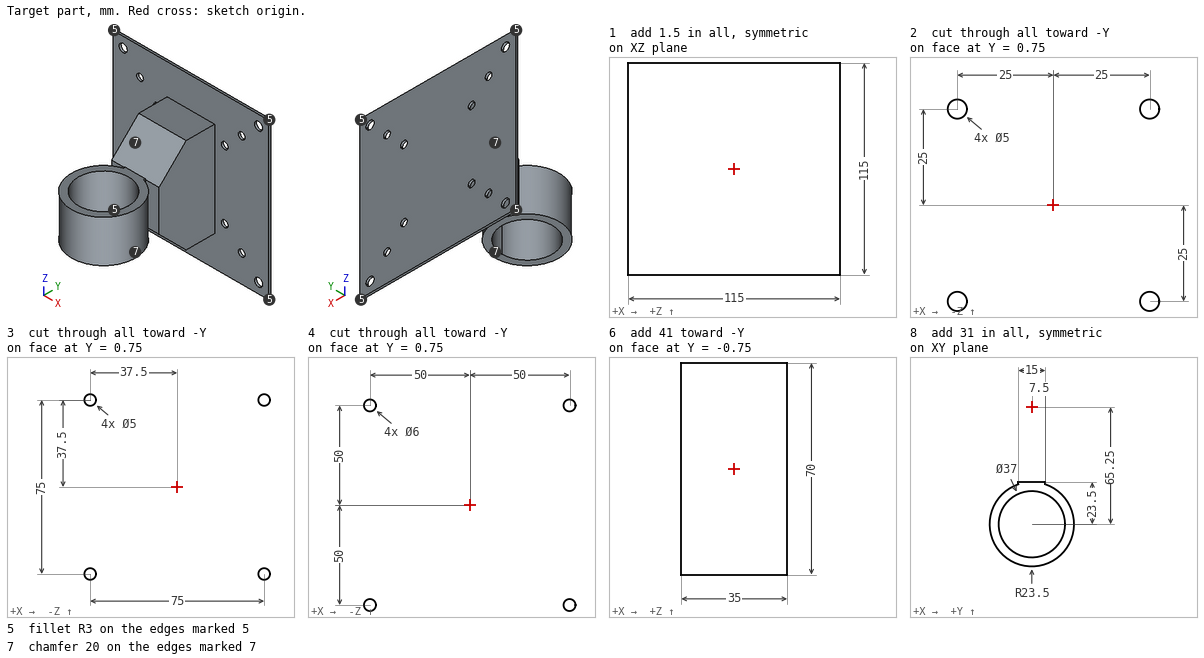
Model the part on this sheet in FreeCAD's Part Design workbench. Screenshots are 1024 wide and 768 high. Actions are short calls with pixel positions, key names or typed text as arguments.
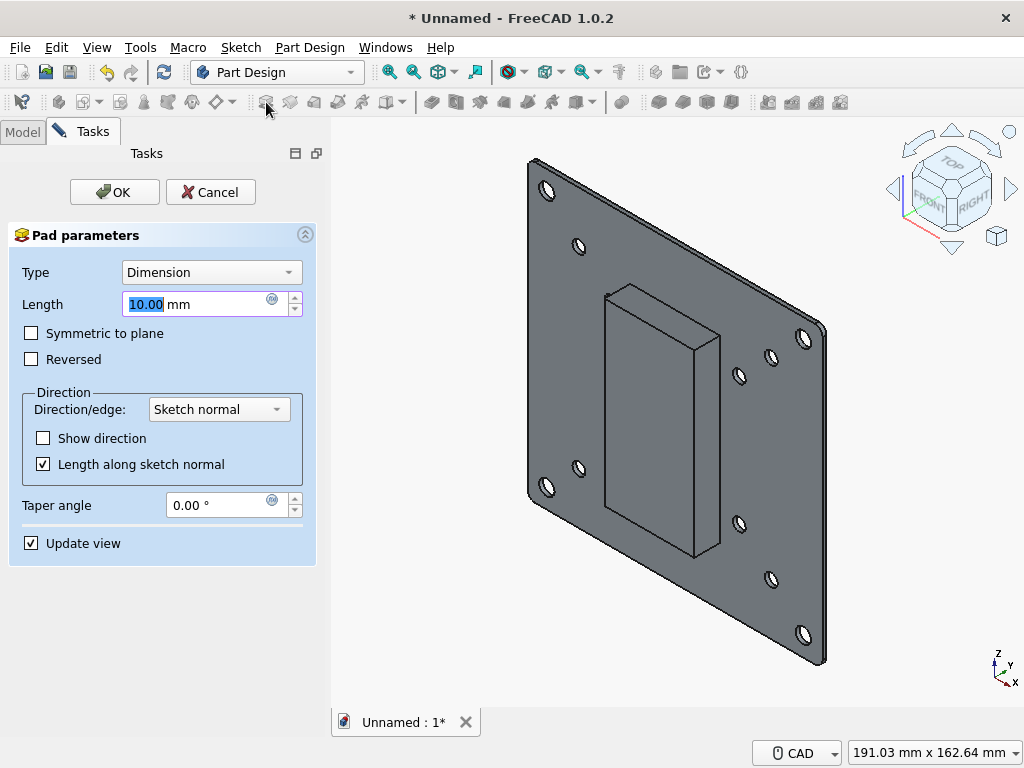
text(41)
key(Tab)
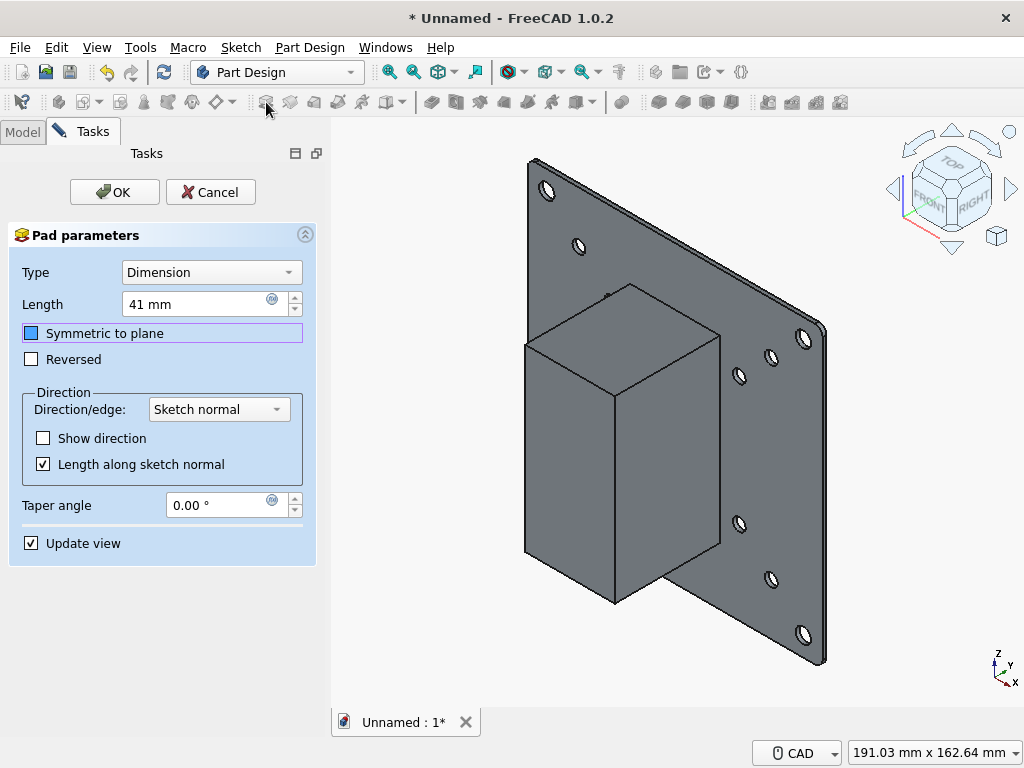
click(115, 192)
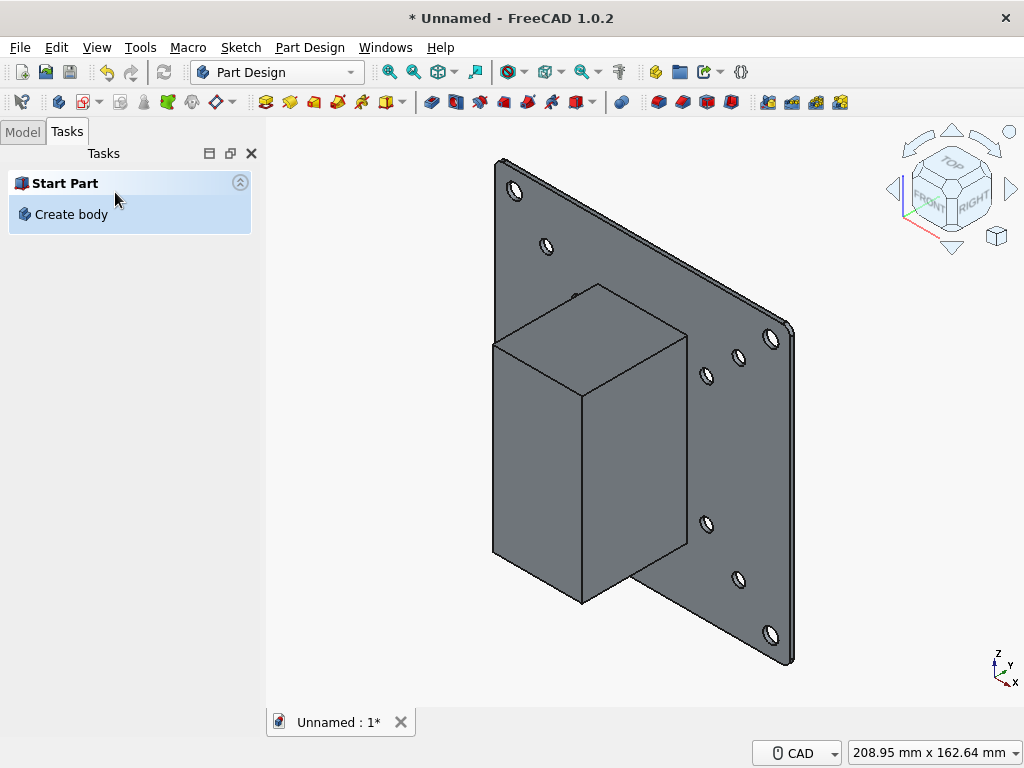
key(v)
key(f)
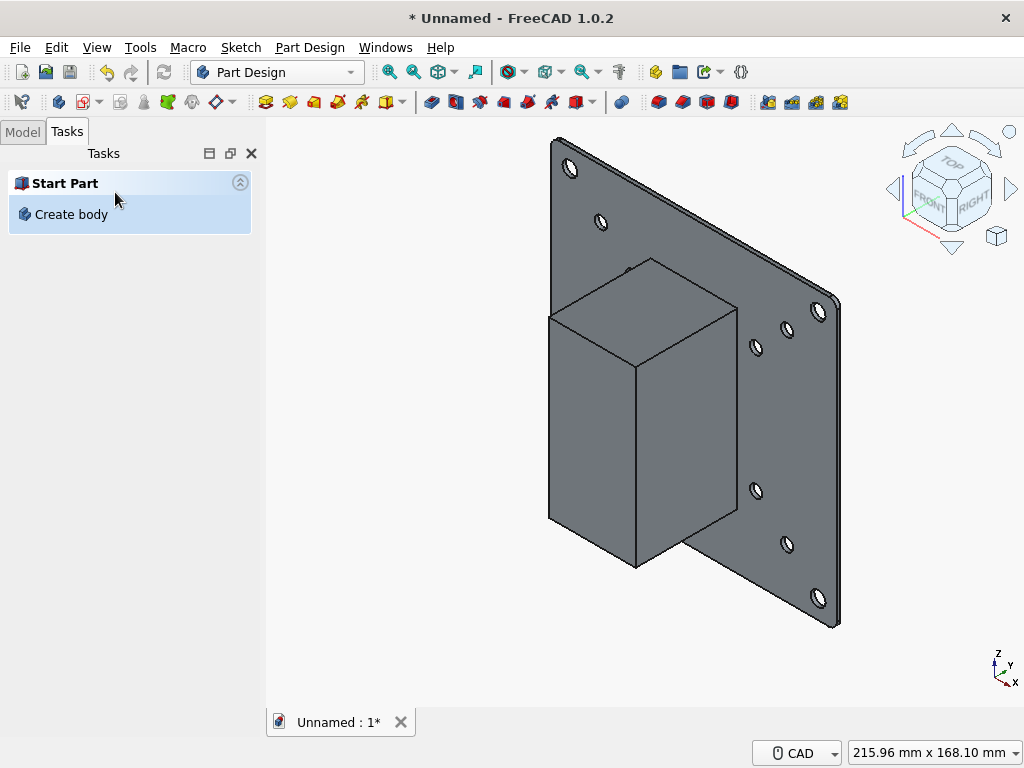
click(592, 341)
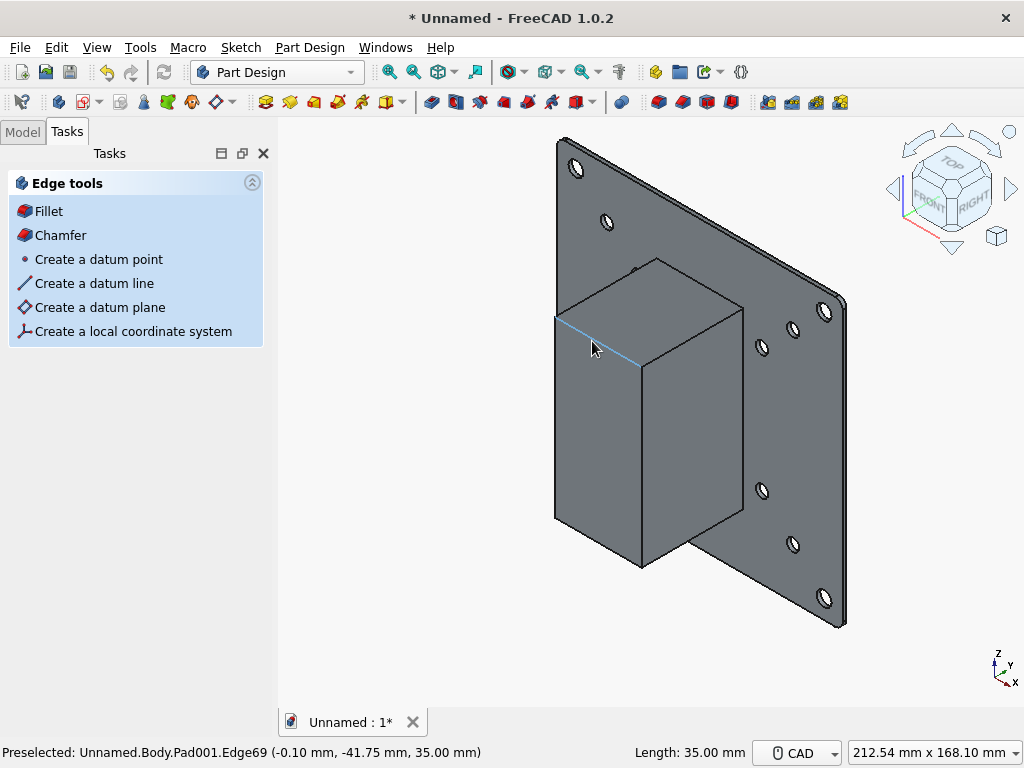
key(2)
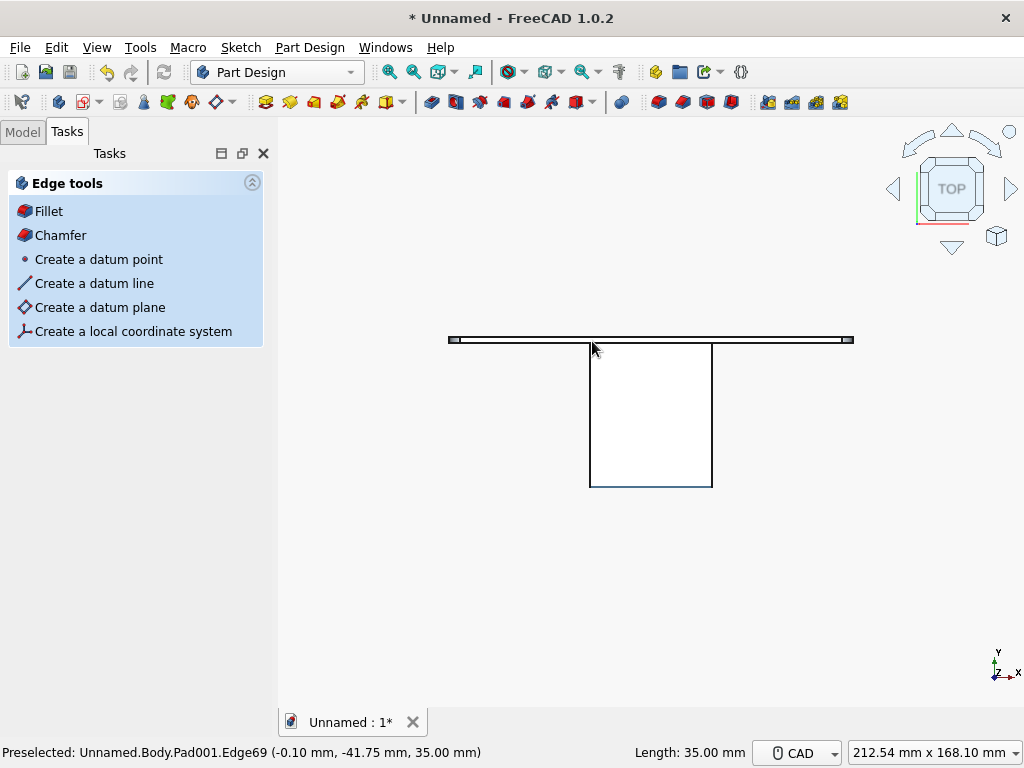
key(0)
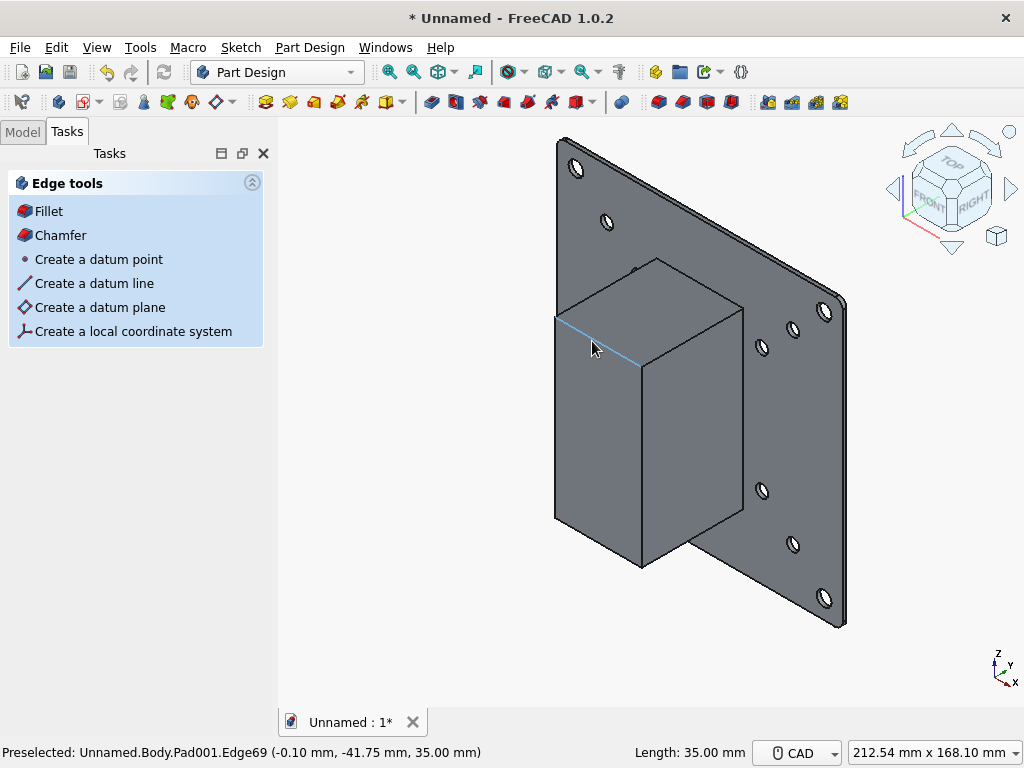
key(1)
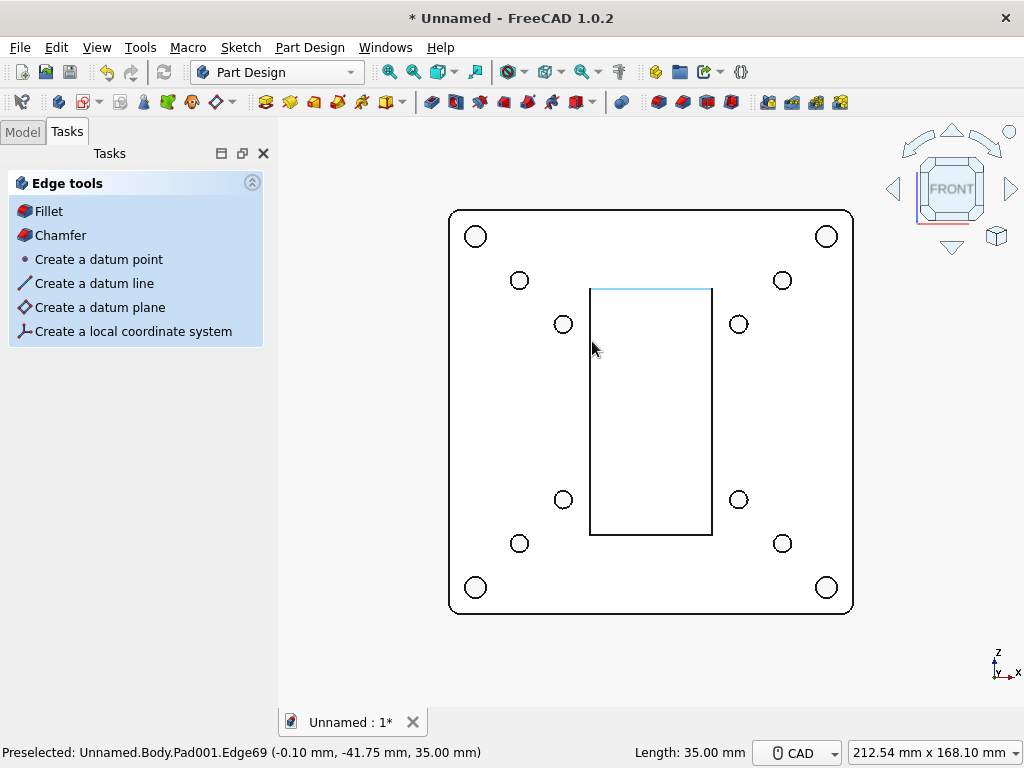
key(3)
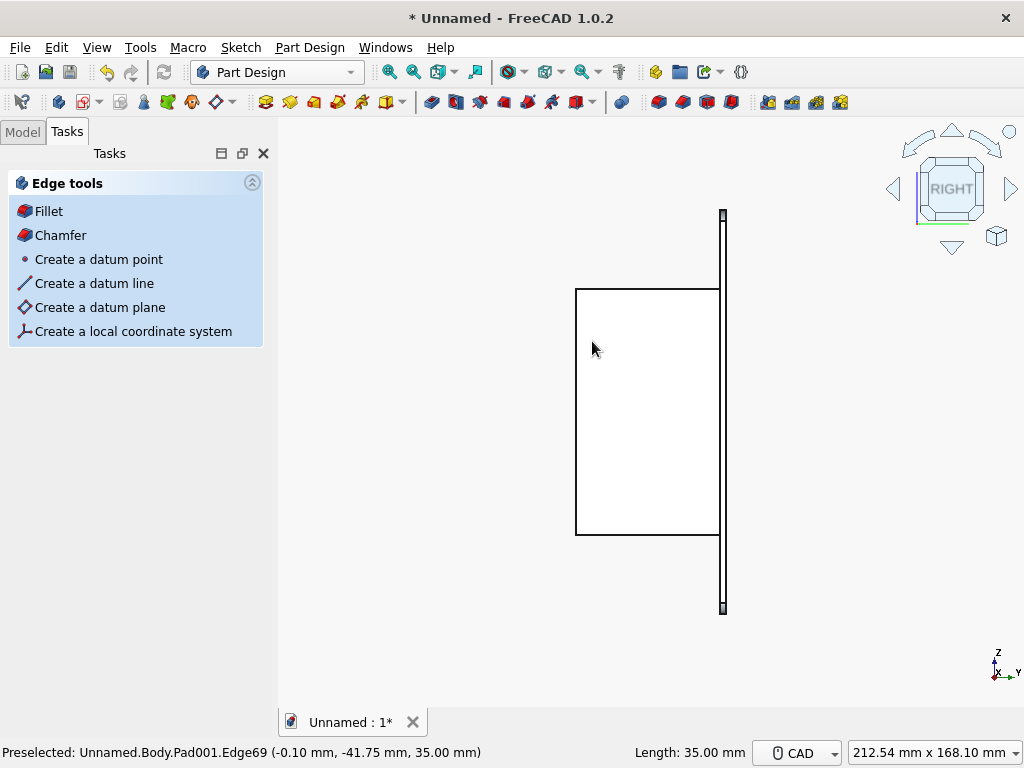
key(5)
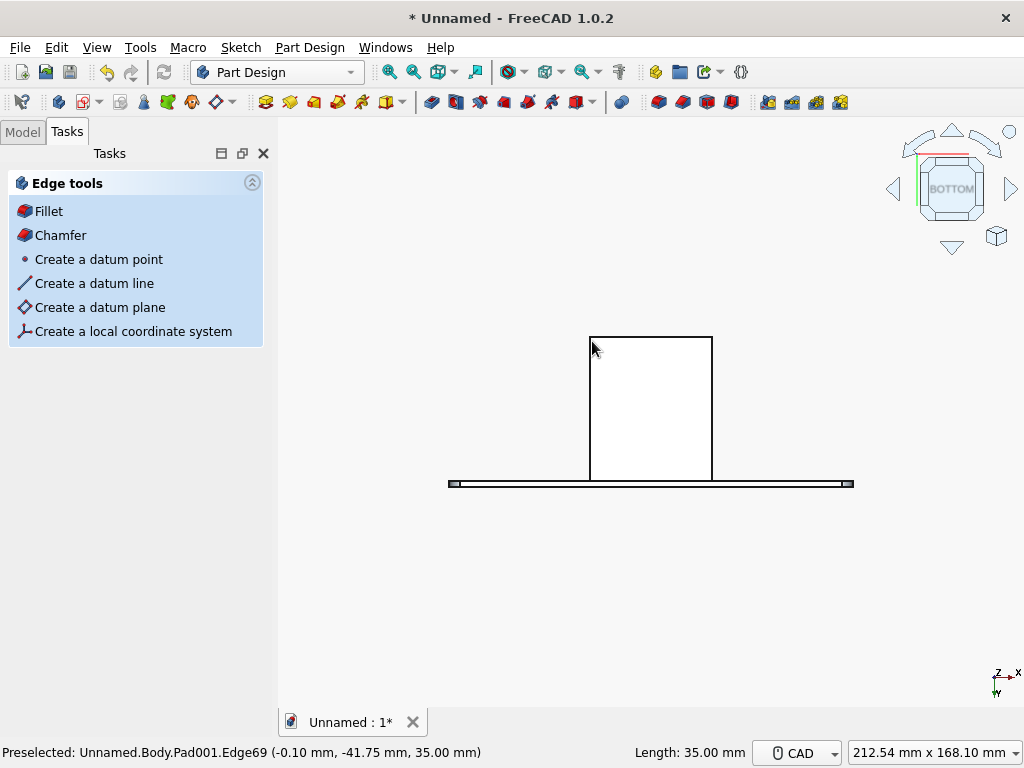
click(651, 336, ctrl)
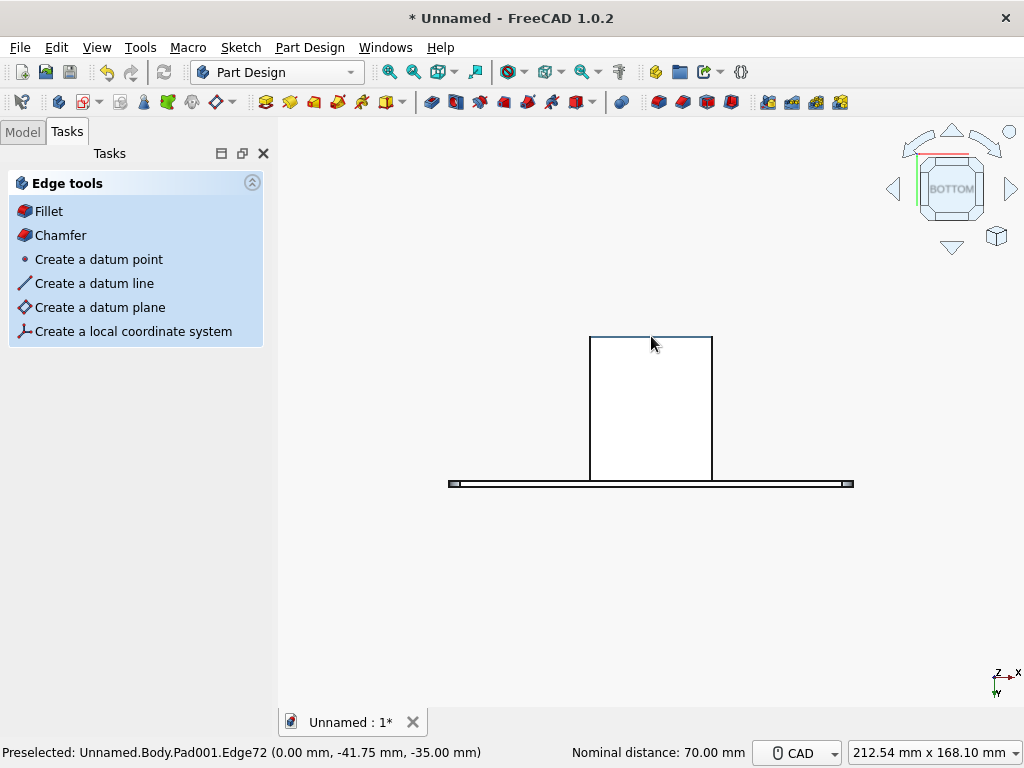
click(684, 102)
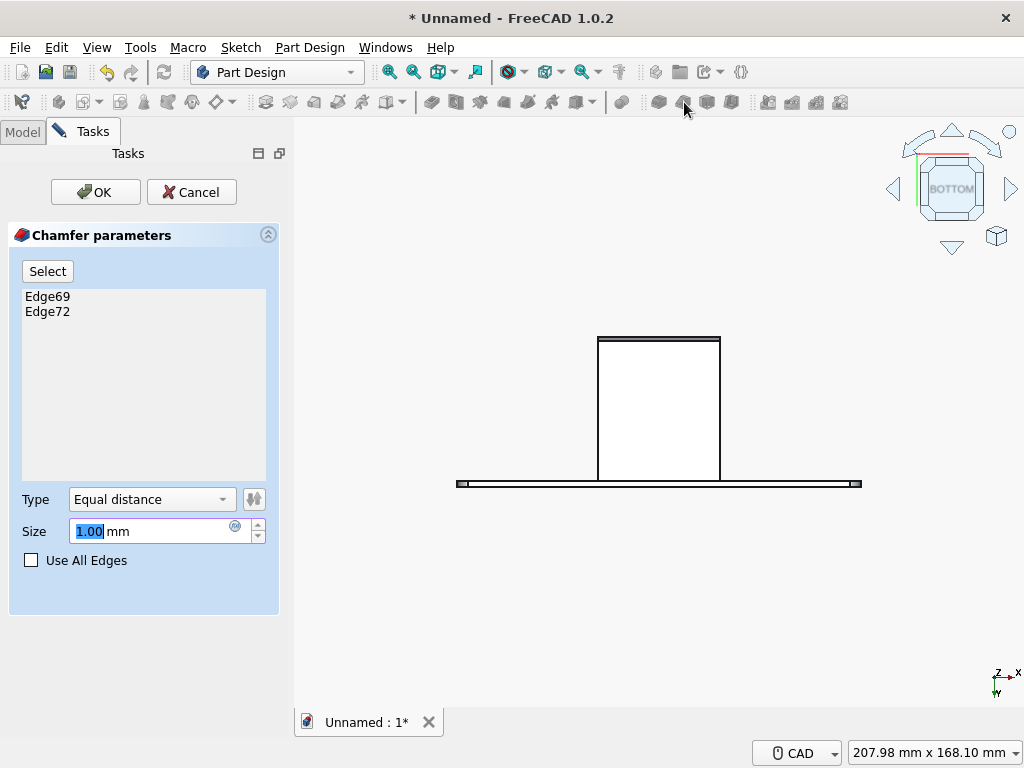
text(20)
key(Tab)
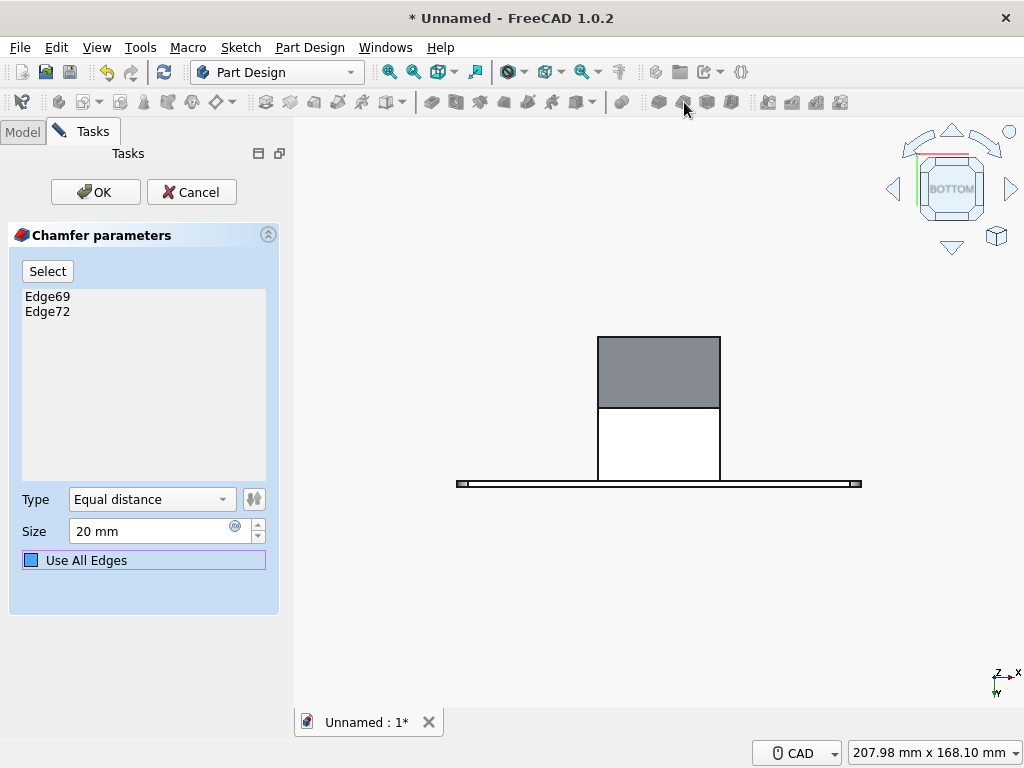
click(96, 192)